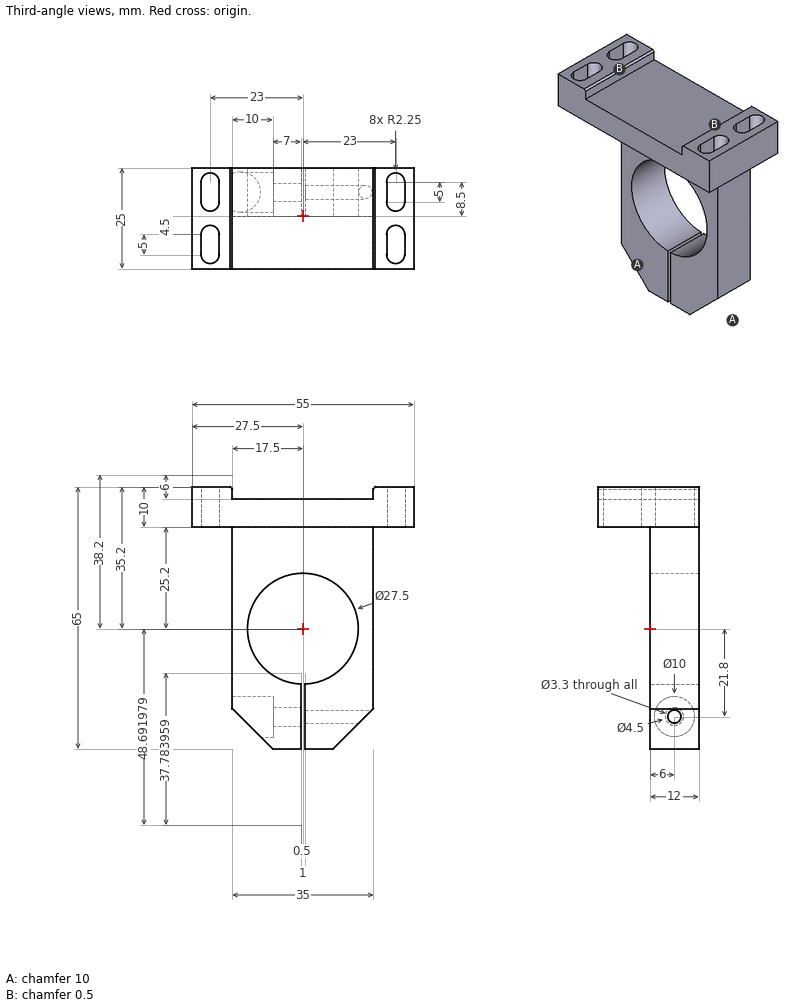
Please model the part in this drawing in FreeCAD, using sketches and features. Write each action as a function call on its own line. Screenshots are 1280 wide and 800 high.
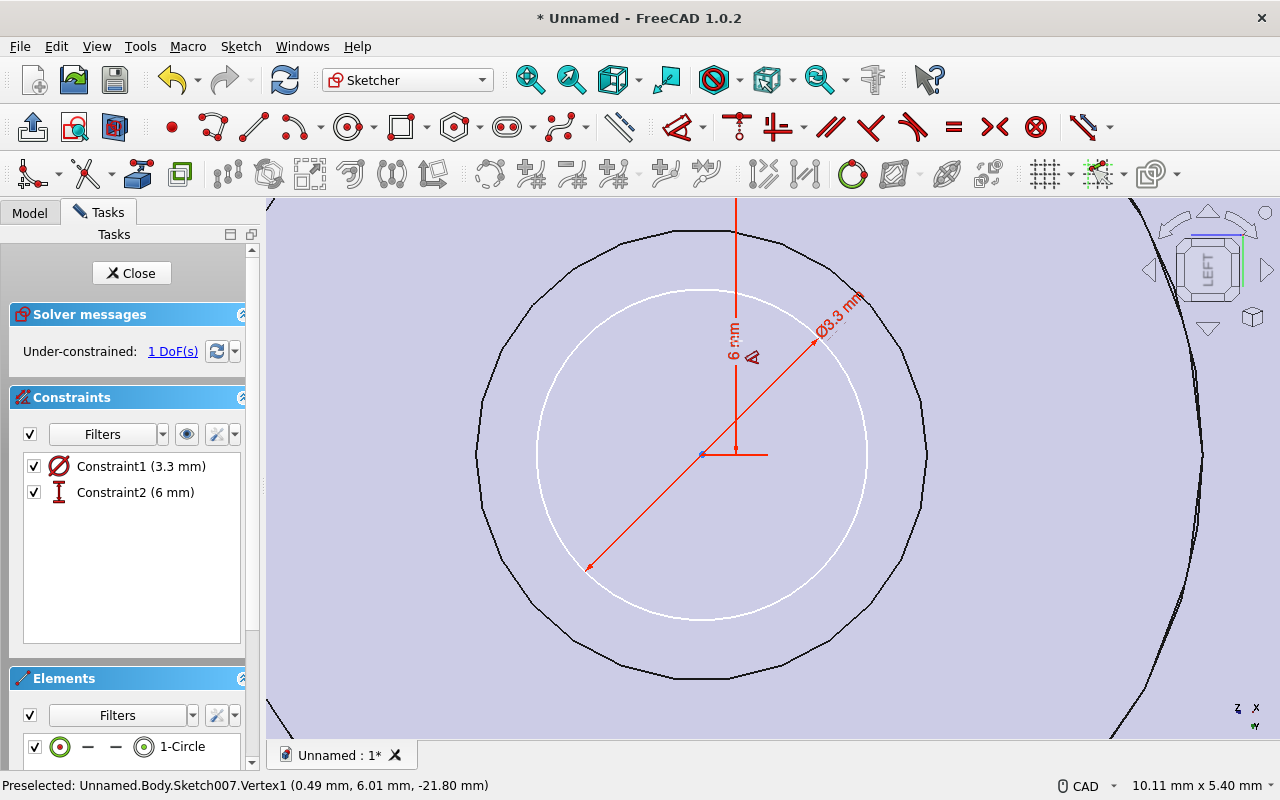
click(702, 455)
click(498, 489)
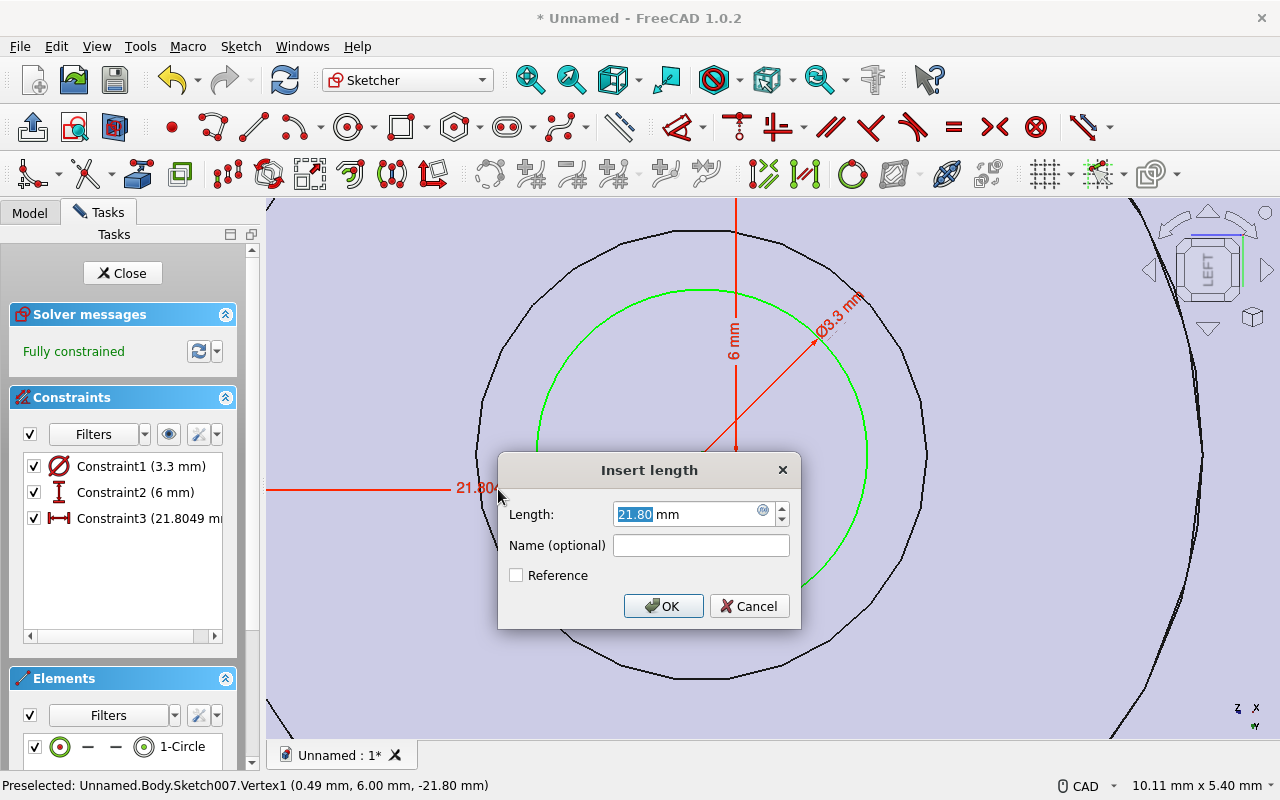
text(21.8)
key(Return)
key(Escape)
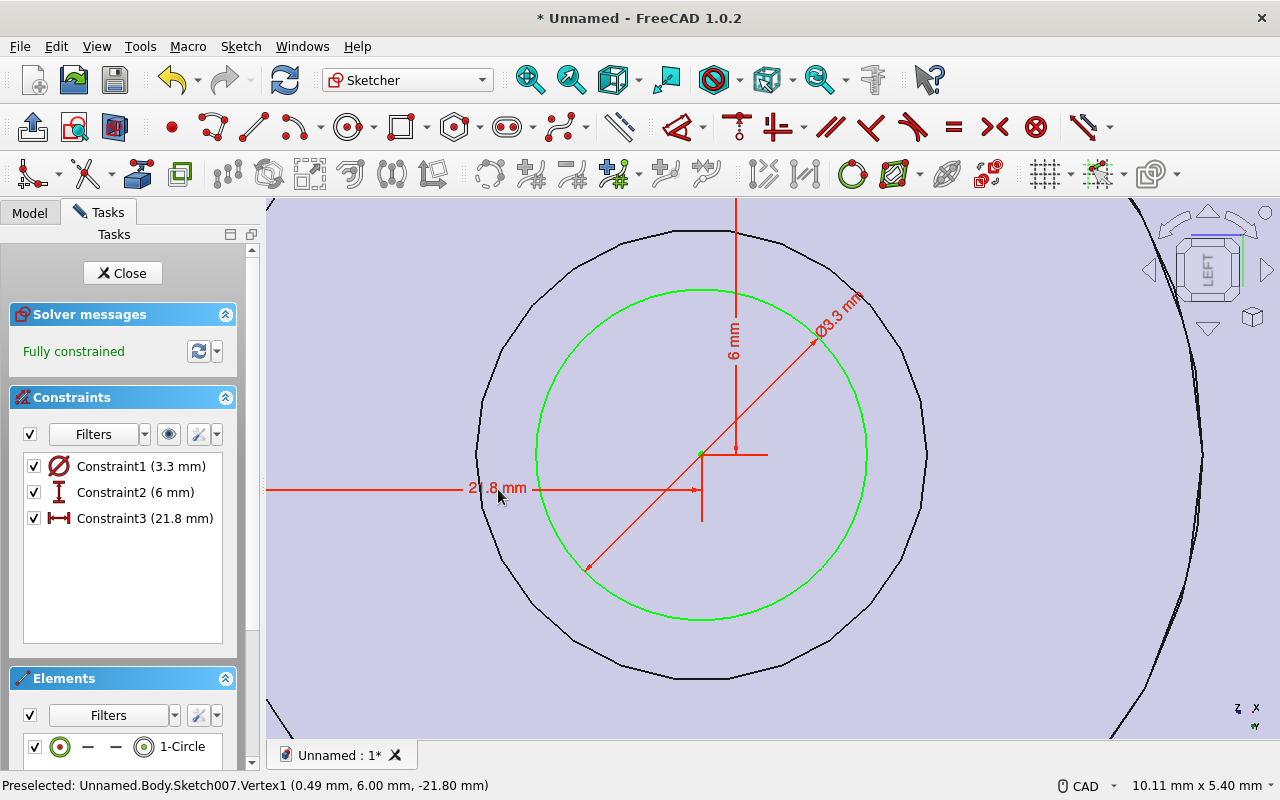
click(123, 273)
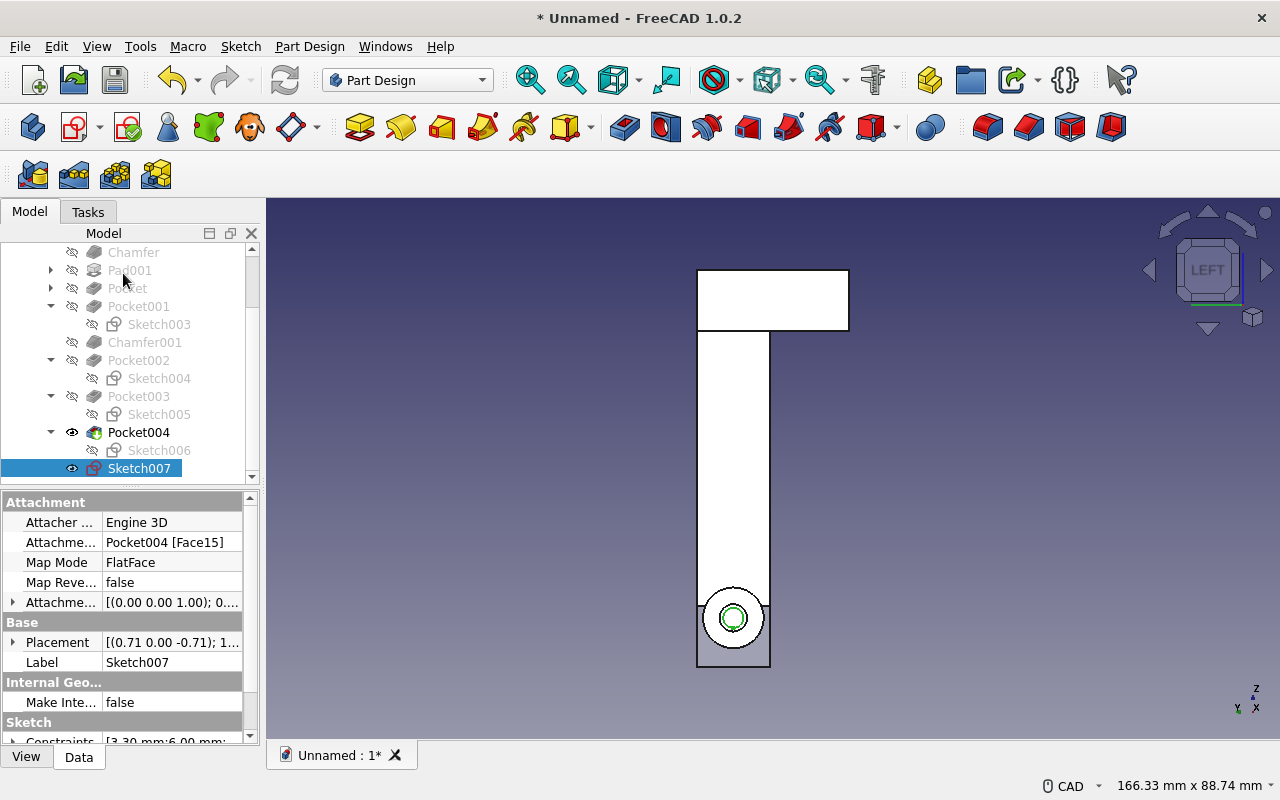
click(666, 128)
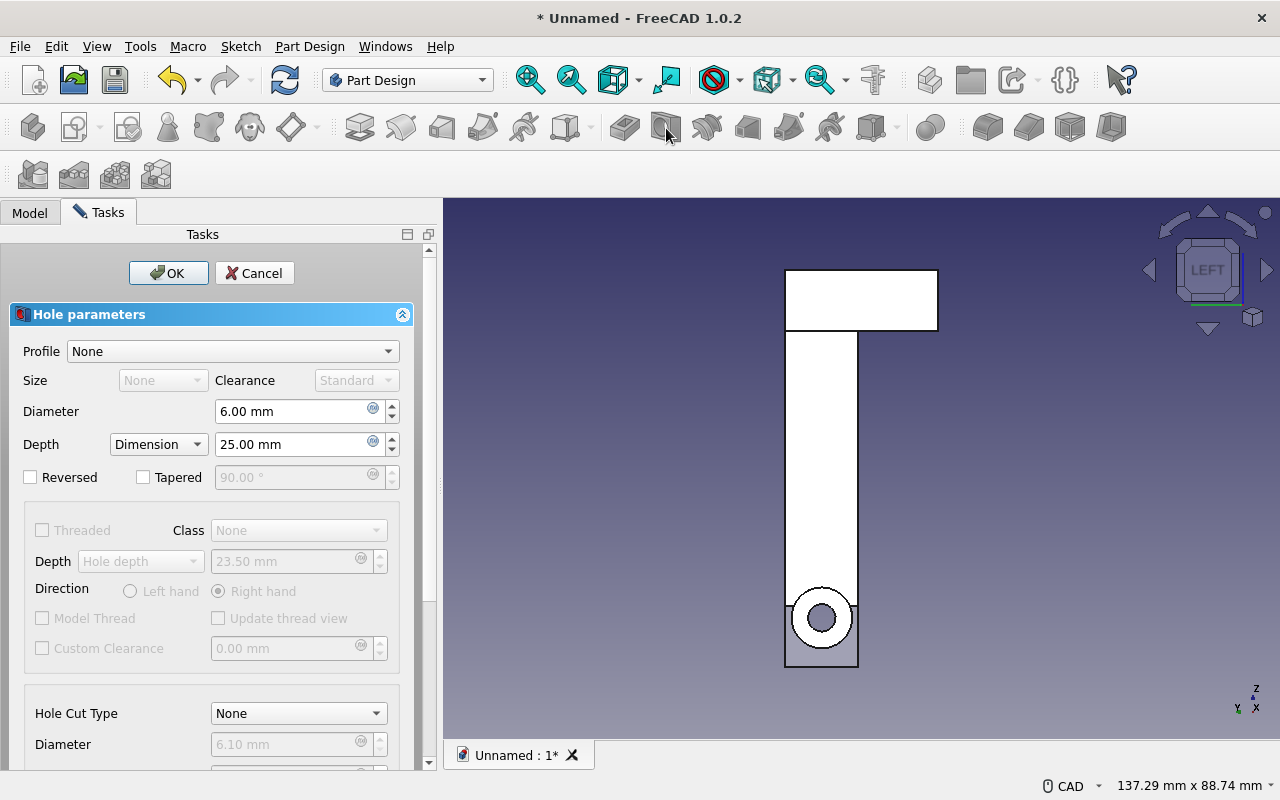
triple_click(300, 412)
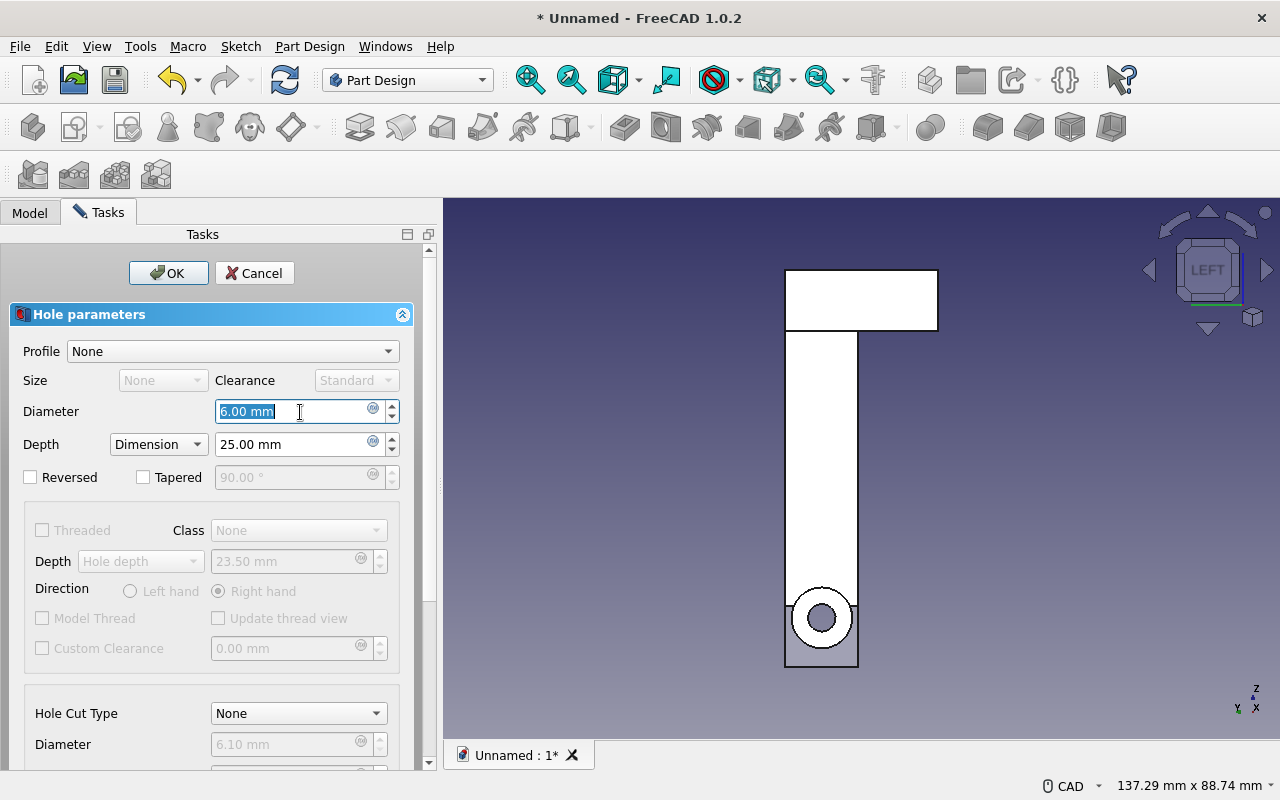
text(3.3)
key(Tab)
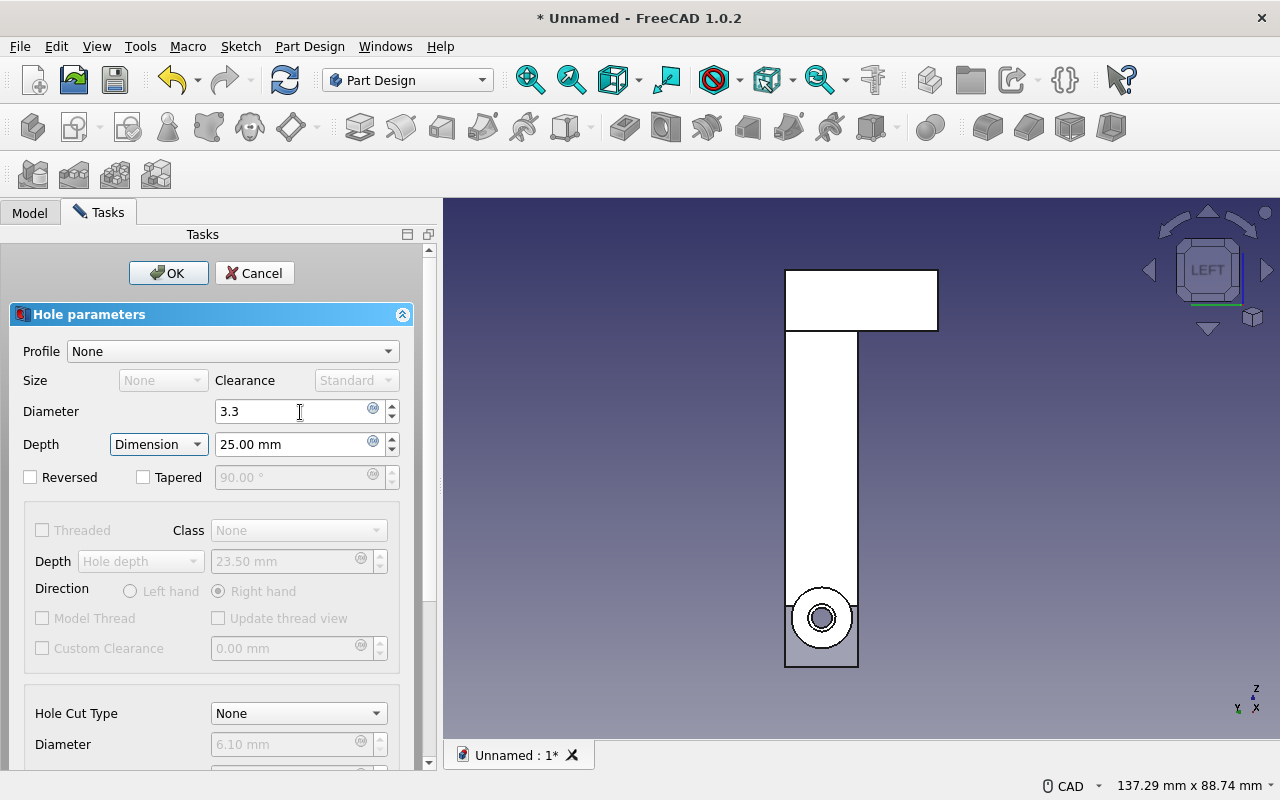
click(160, 444)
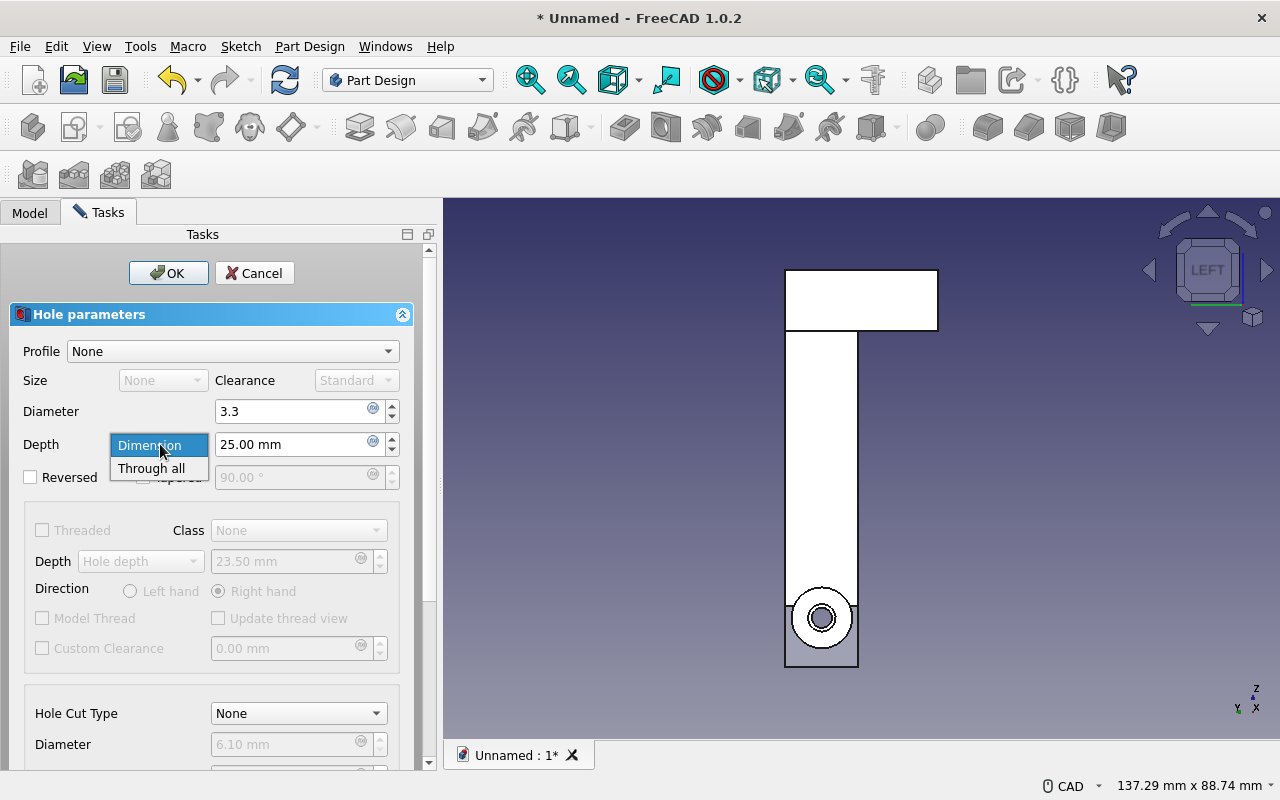
click(158, 468)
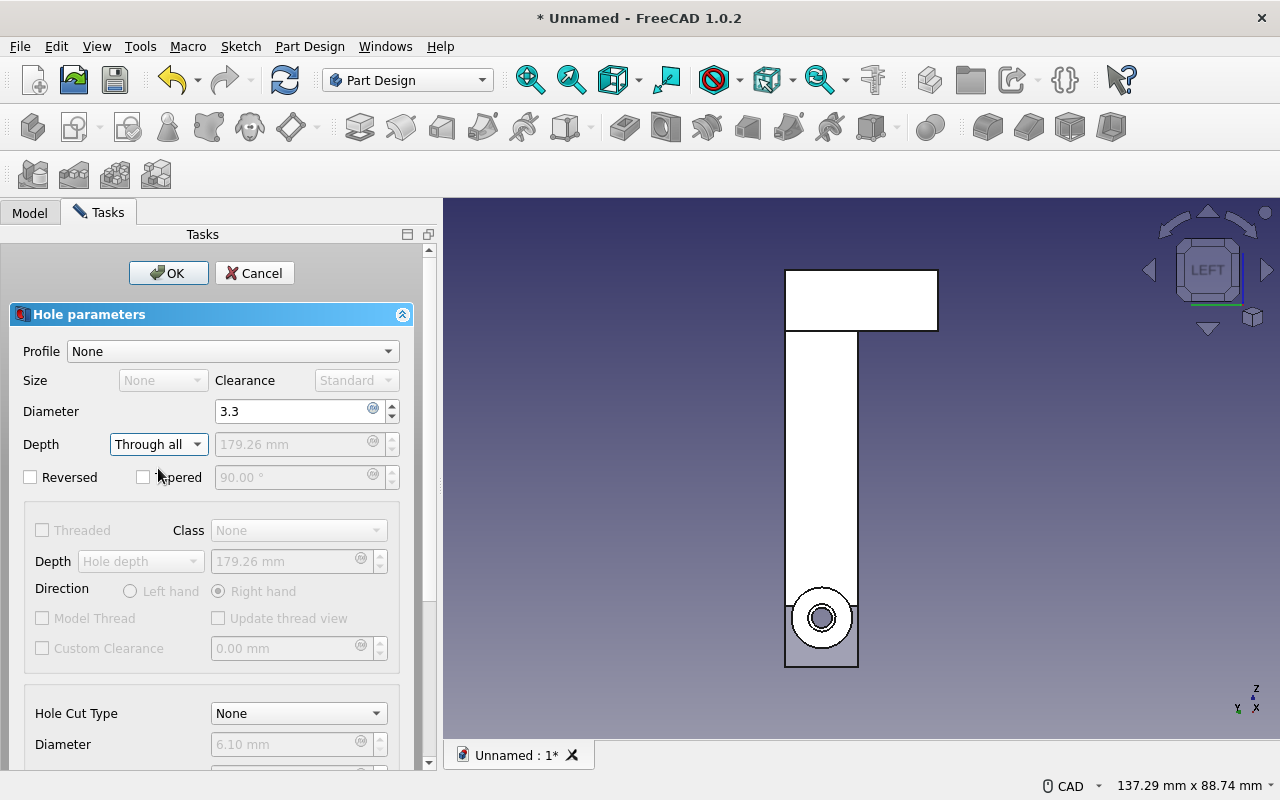
click(169, 273)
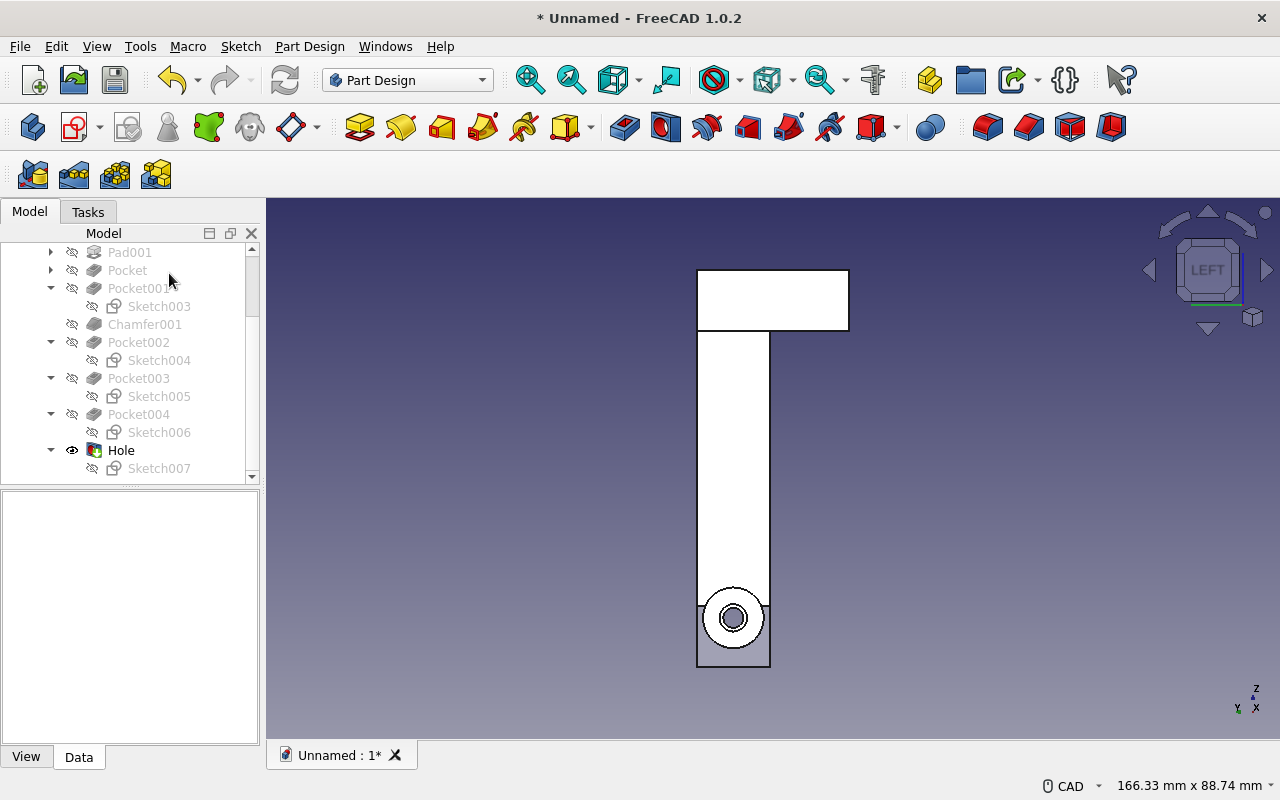
key(0)